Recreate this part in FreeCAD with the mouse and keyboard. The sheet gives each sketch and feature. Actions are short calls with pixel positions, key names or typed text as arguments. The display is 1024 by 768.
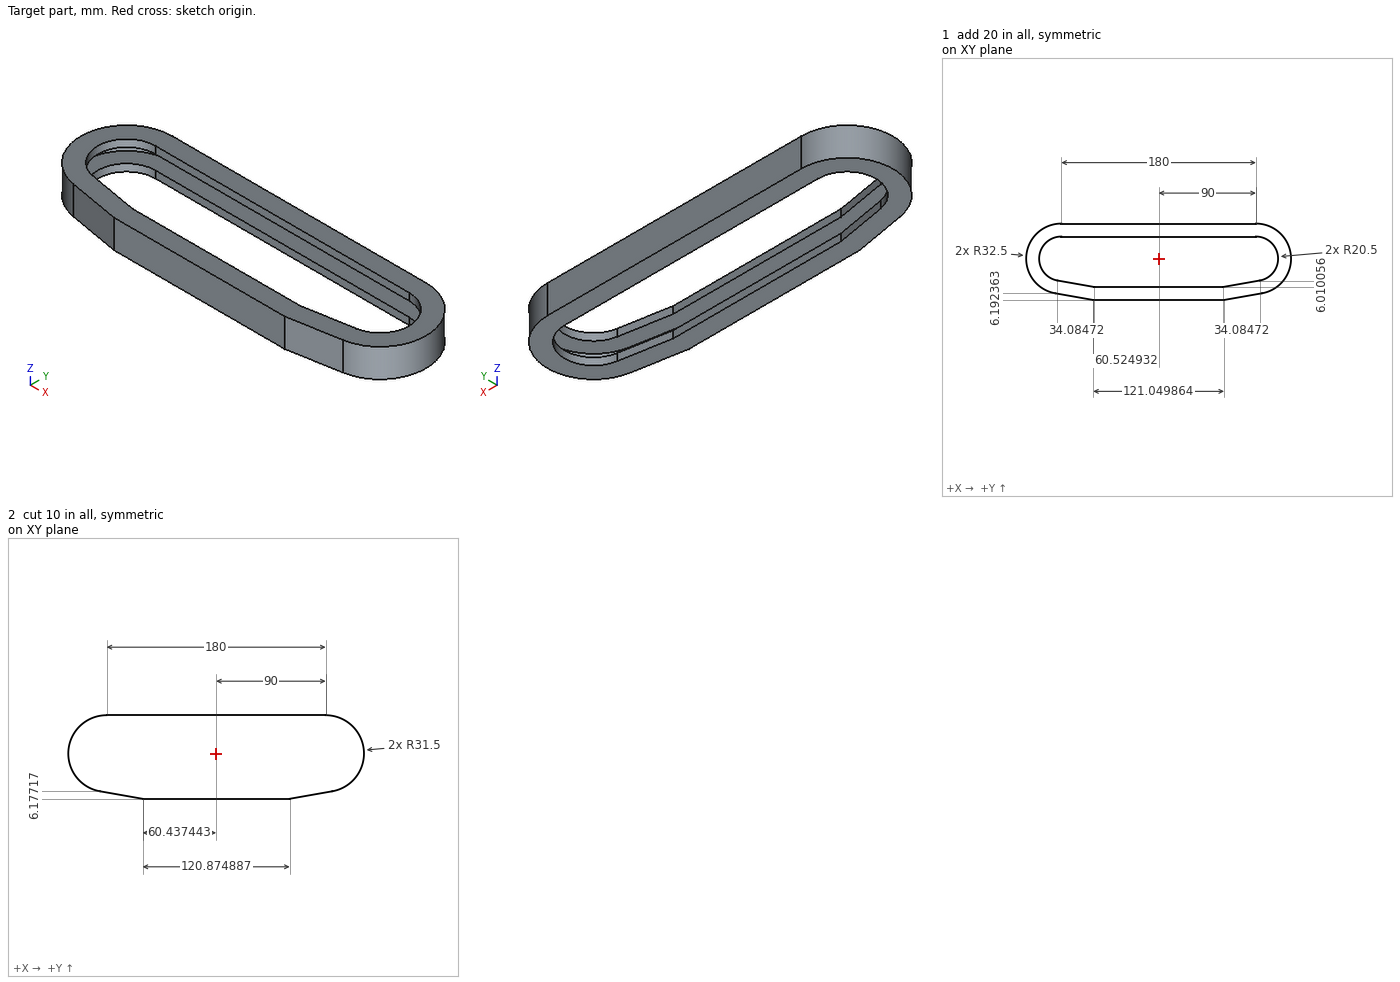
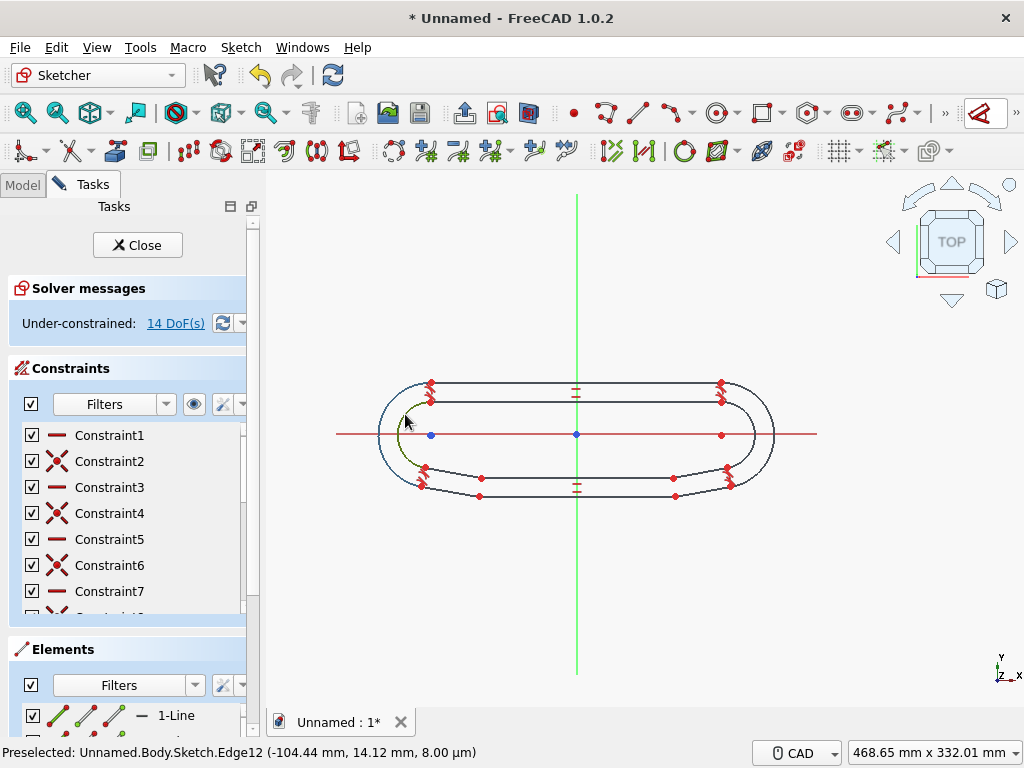
key(c)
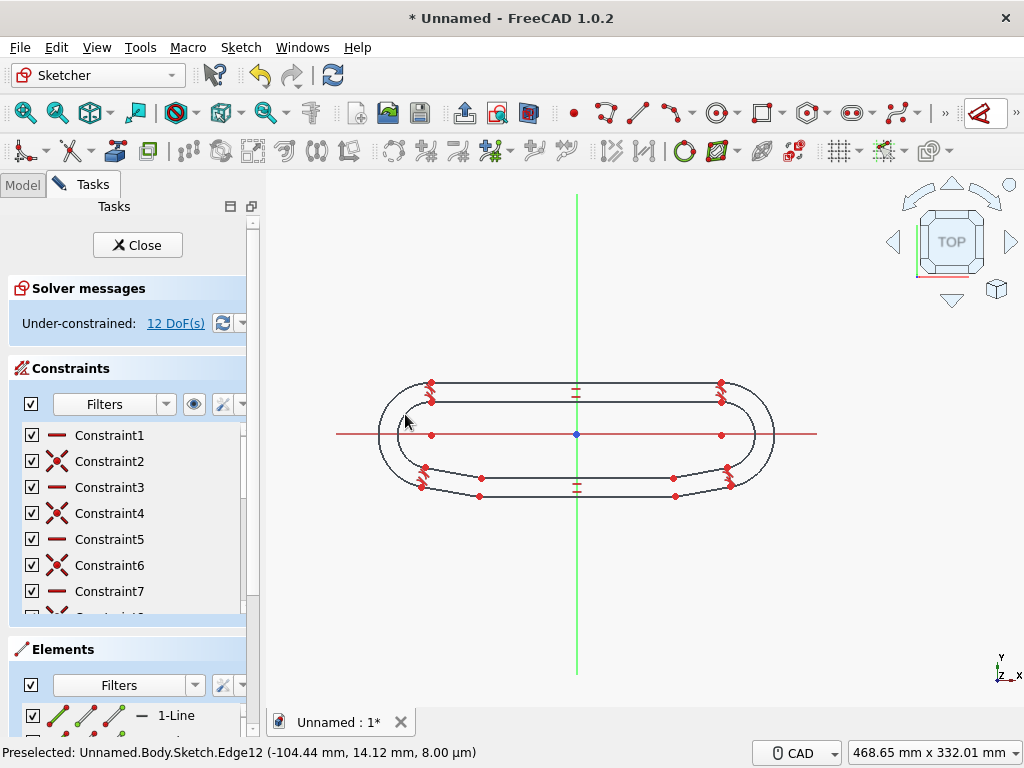
click(390, 402)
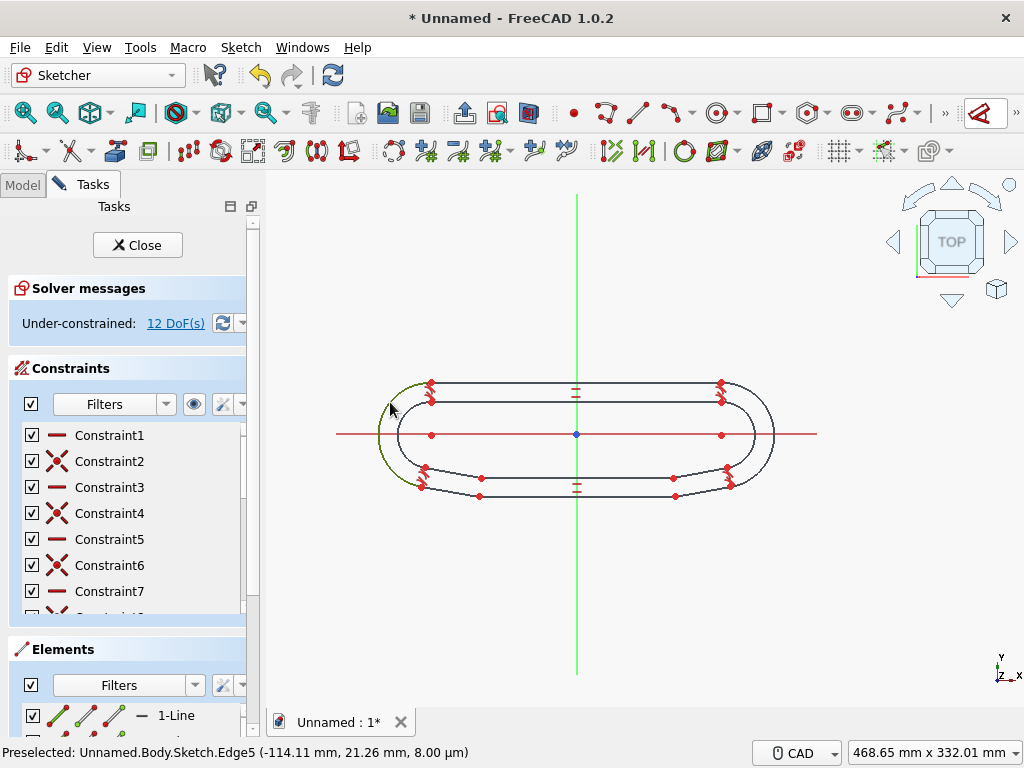
click(768, 461)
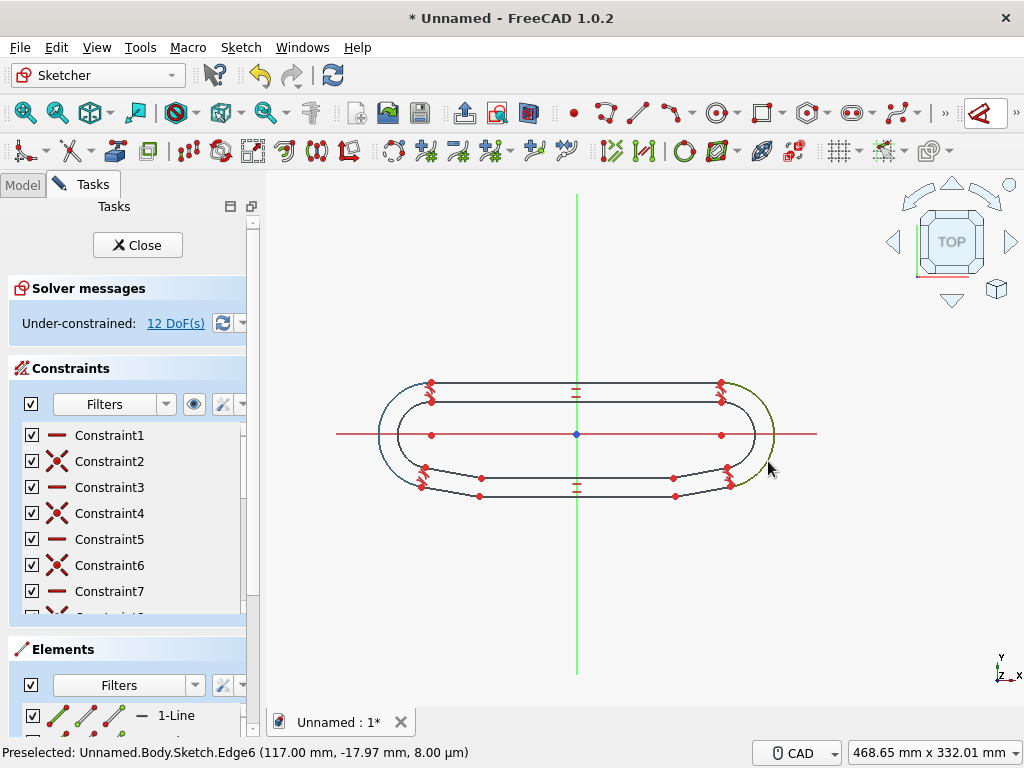
key(e)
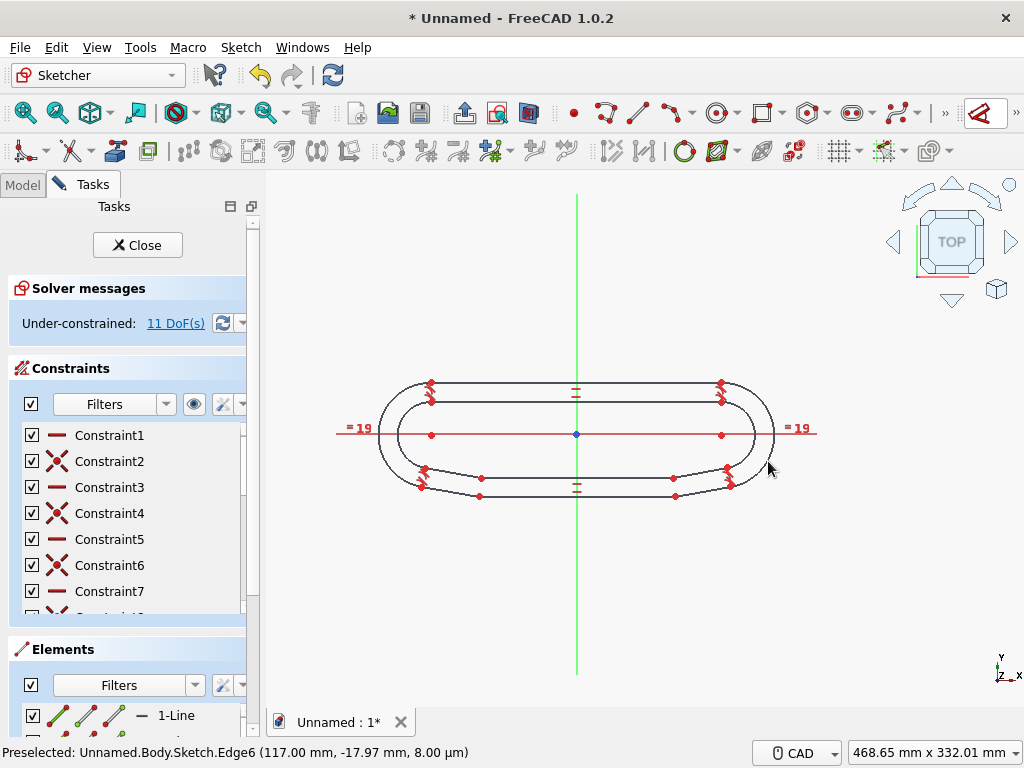
click(431, 435)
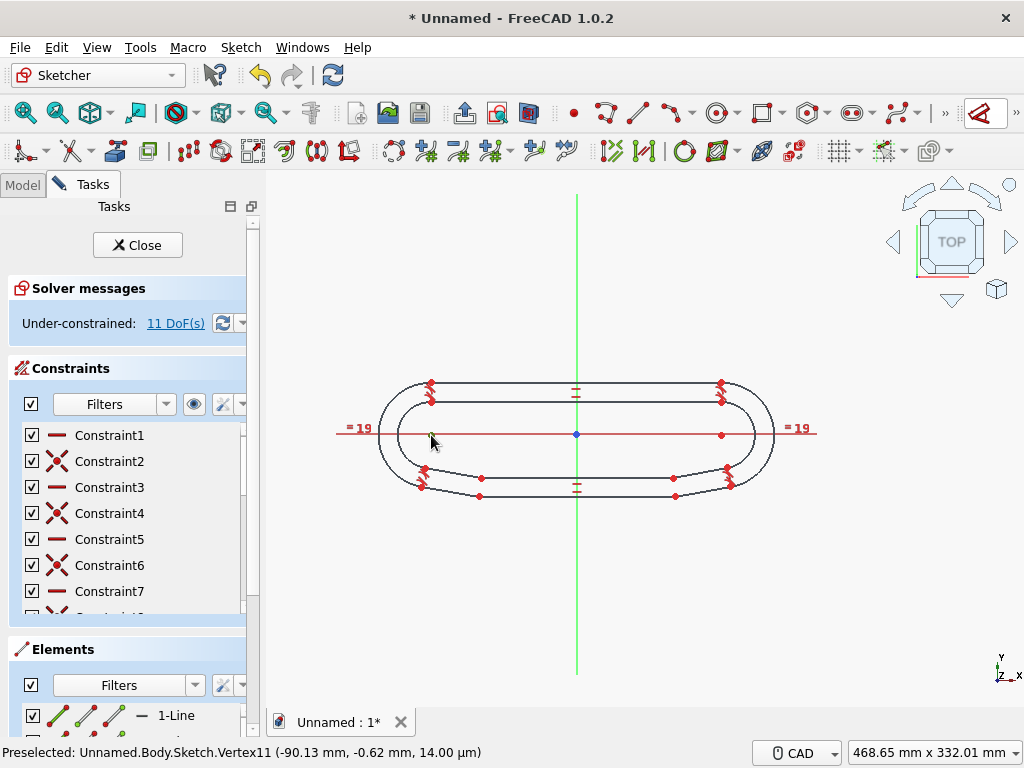
click(334, 434)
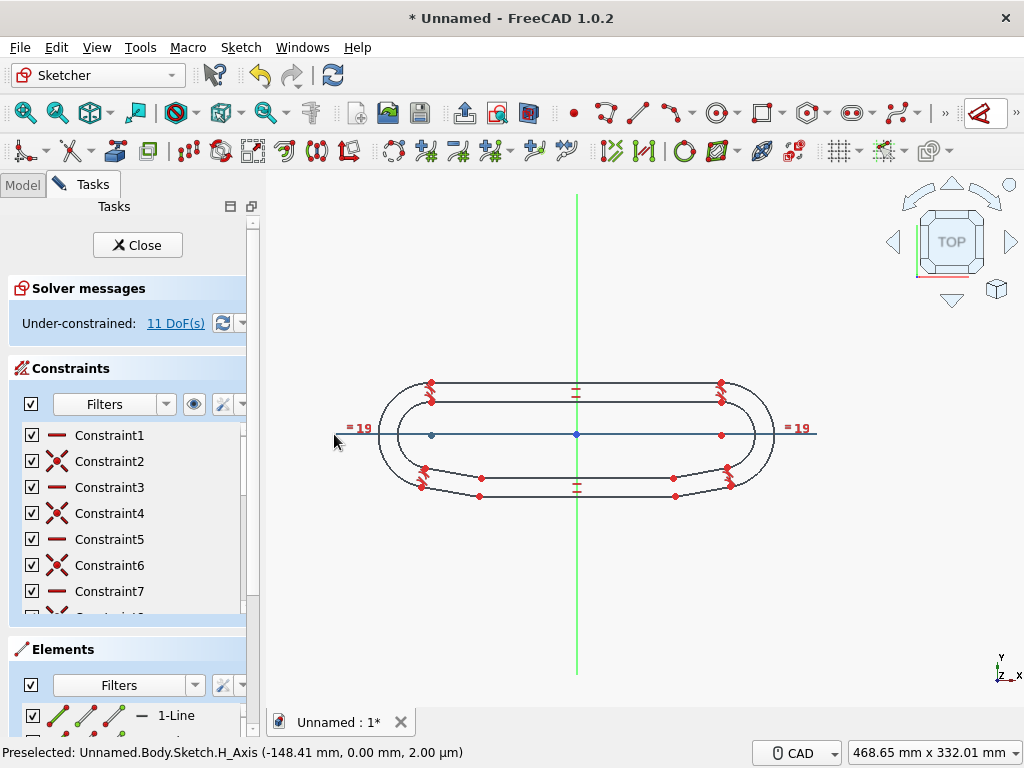
key(c)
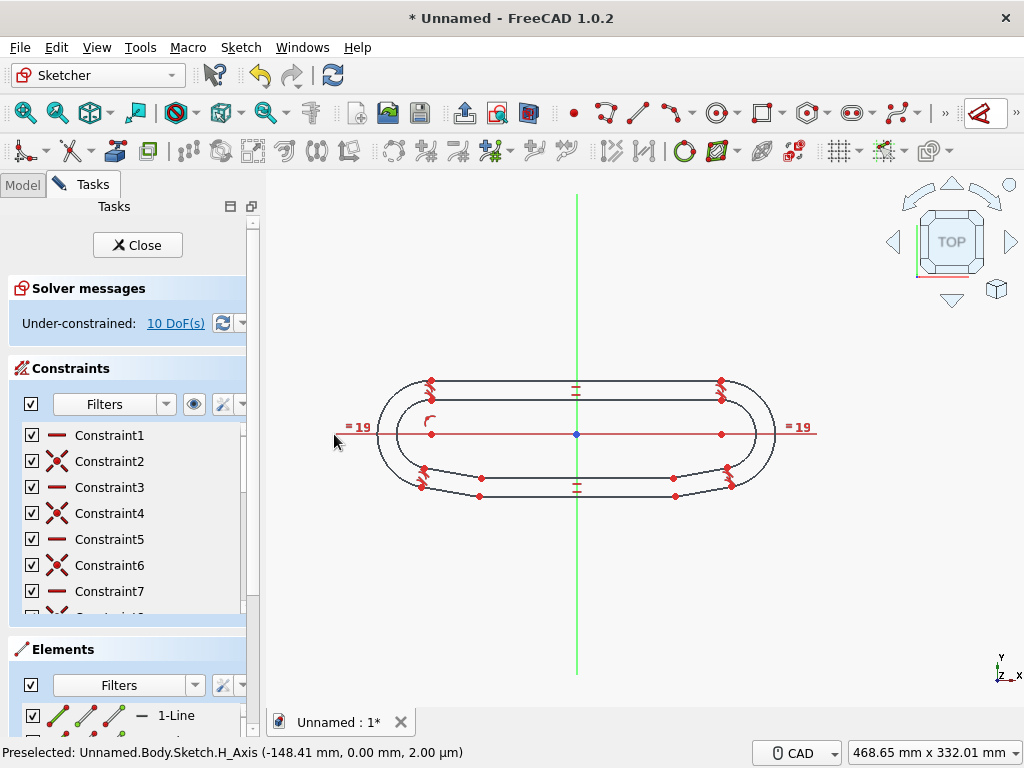
key(d)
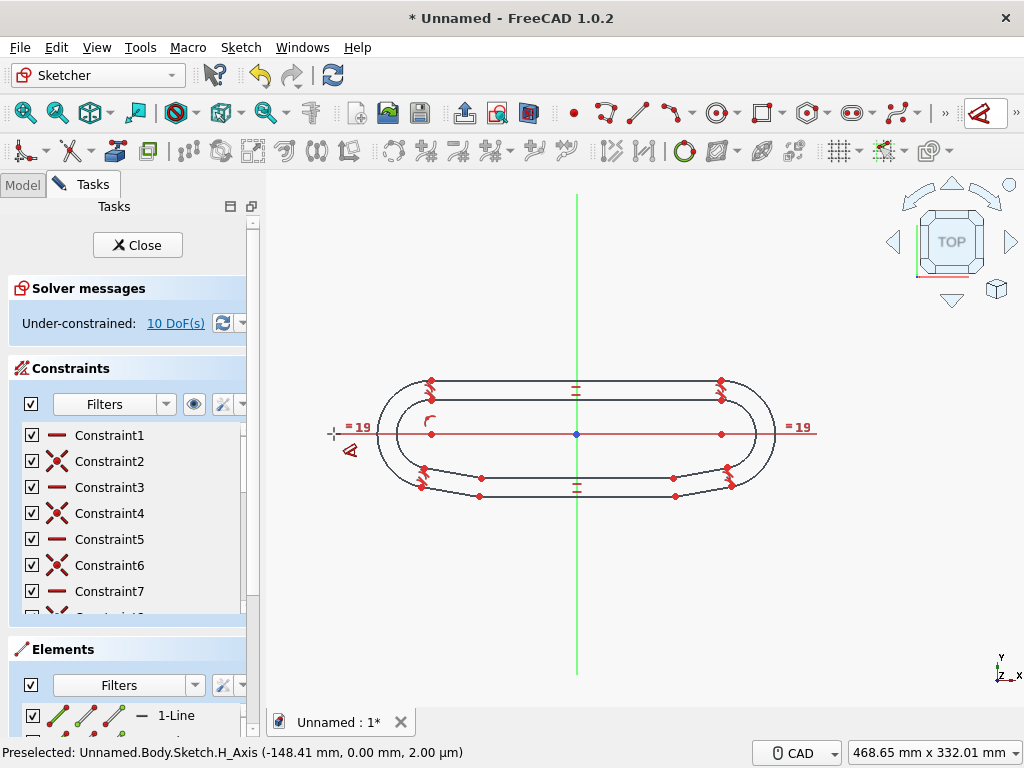
click(389, 401)
click(364, 381)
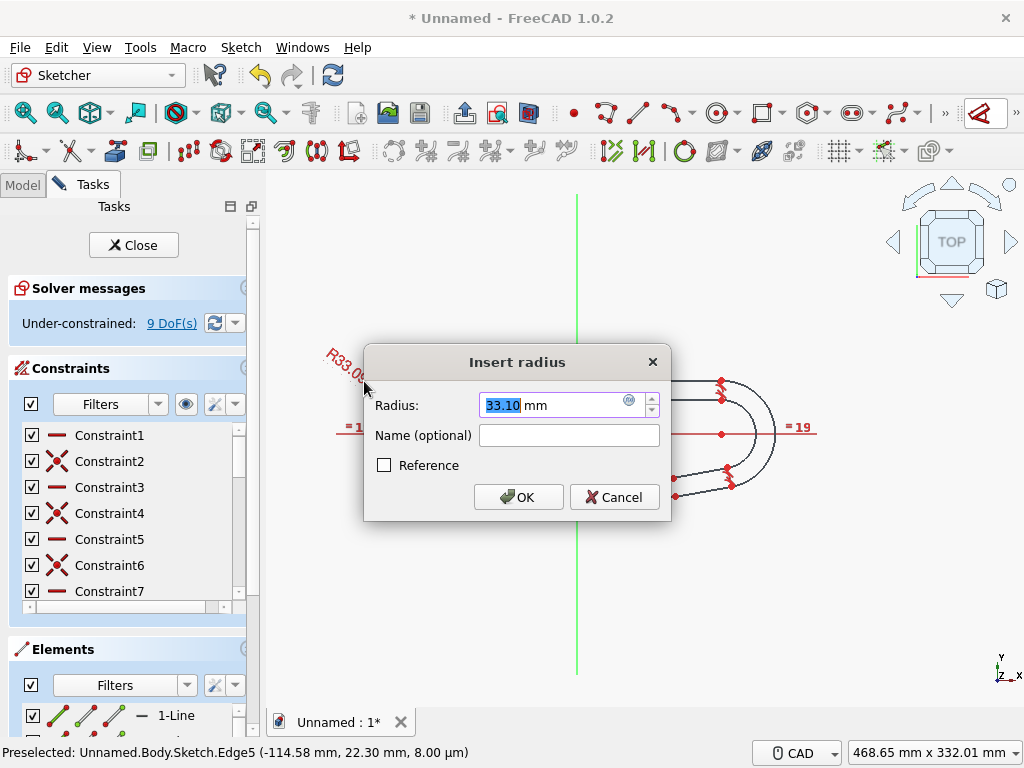
text(32.5)
key(Return)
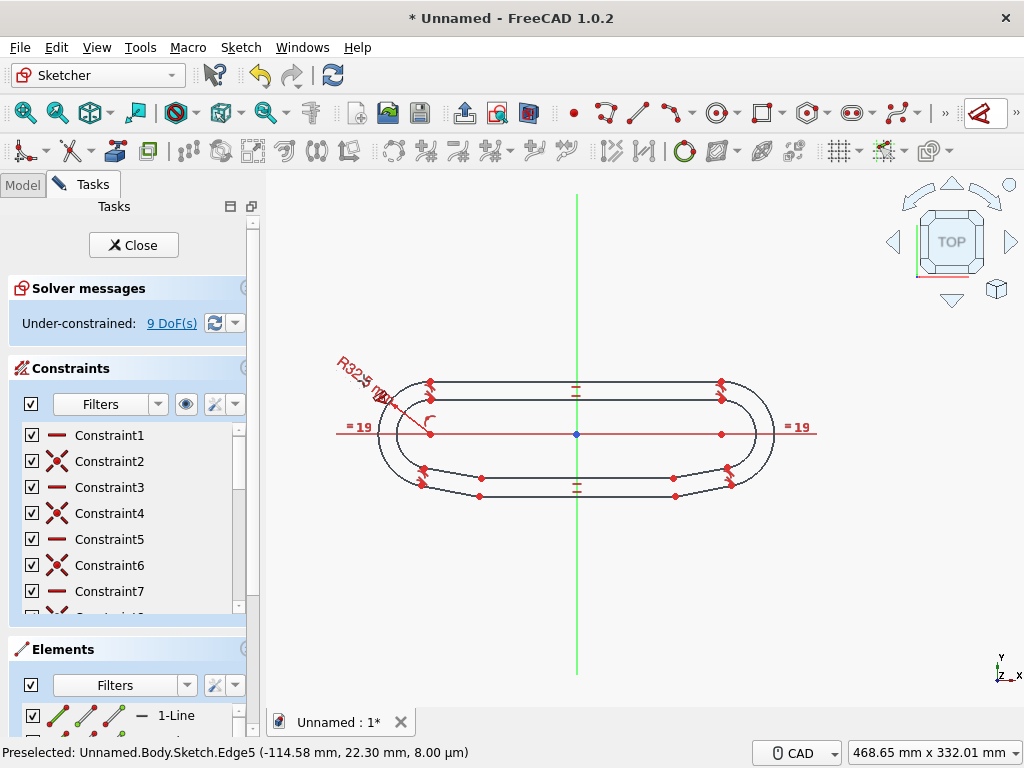
click(752, 451)
click(780, 466)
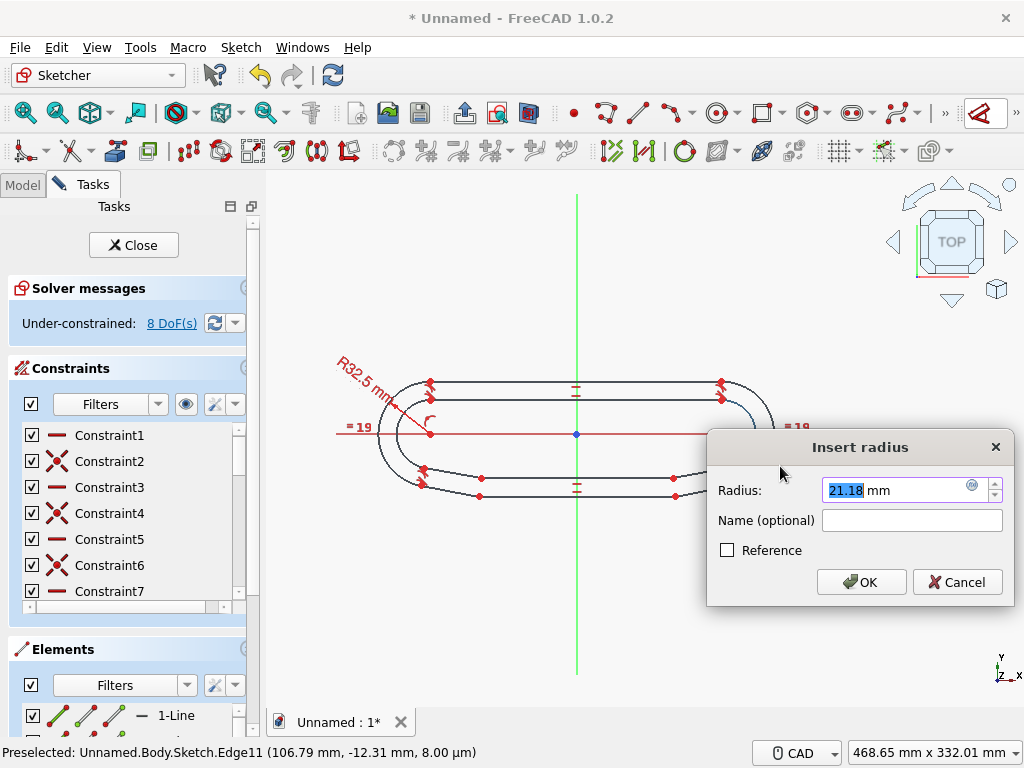
text(20.5)
key(Return)